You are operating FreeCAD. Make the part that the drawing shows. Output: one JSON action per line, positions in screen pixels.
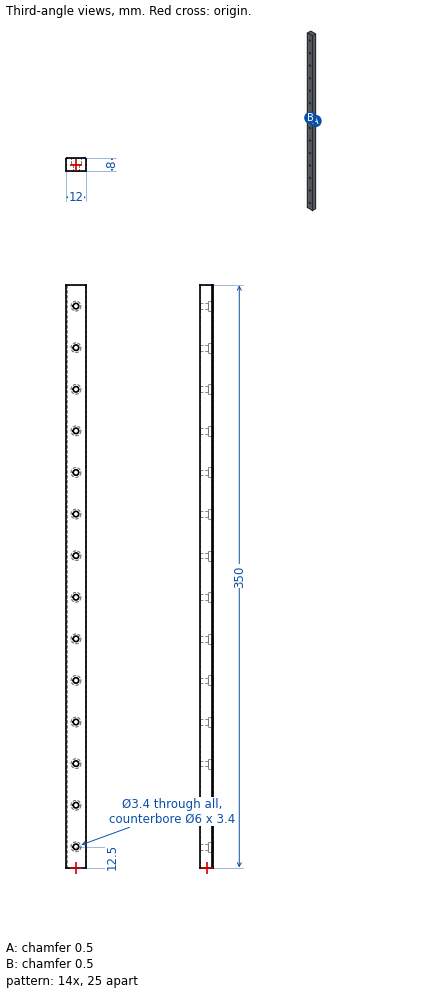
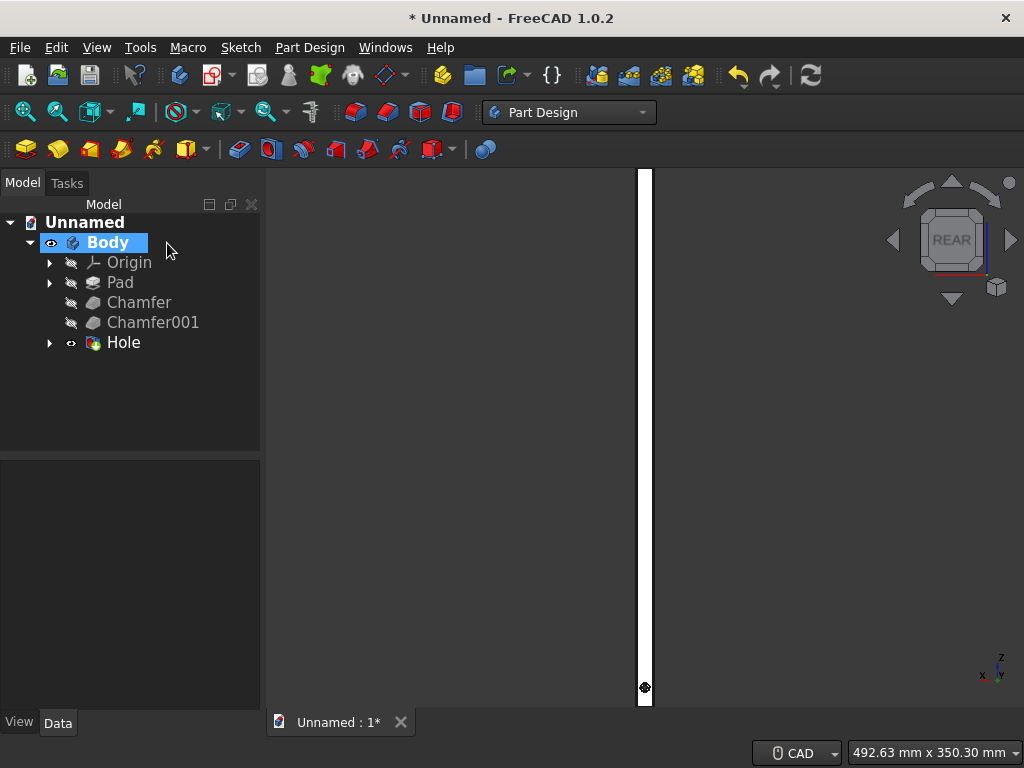
{"action": "left_click", "coordinate": [26, 112]}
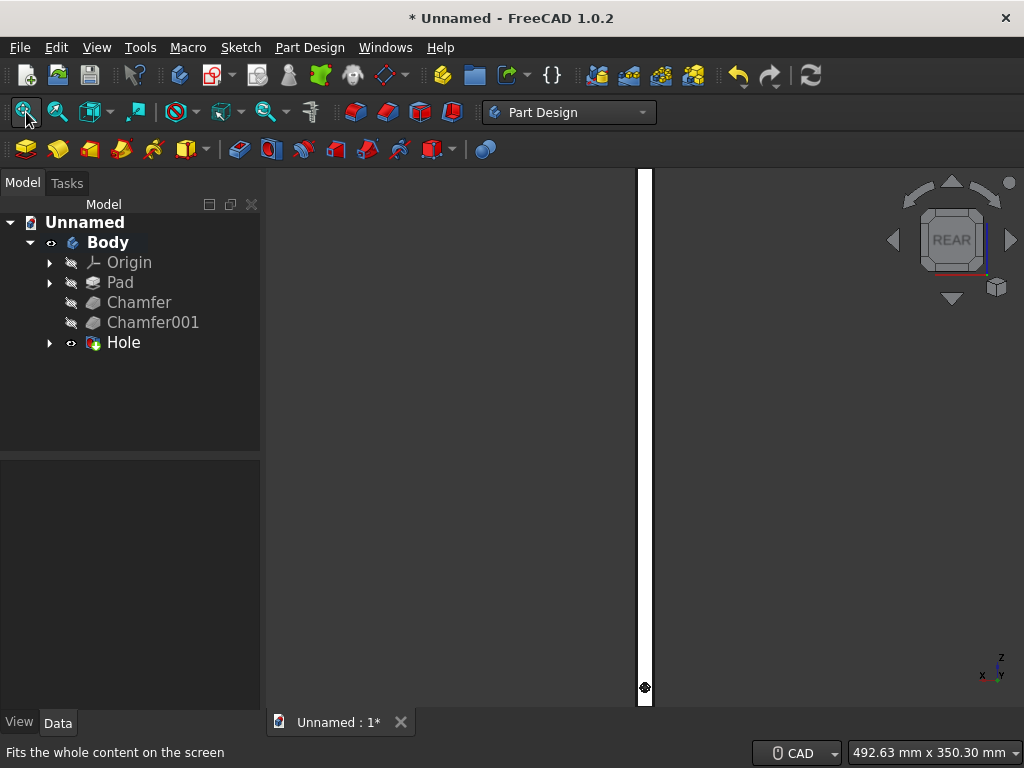
{"action": "left_click", "coordinate": [116, 343]}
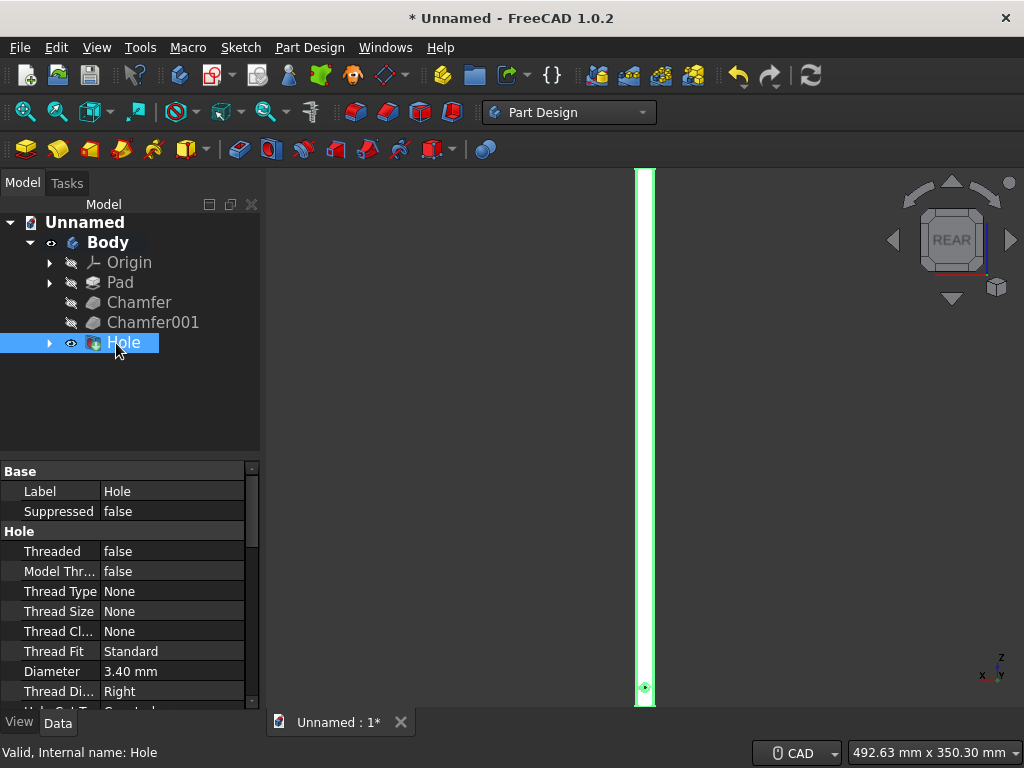
{"action": "left_click", "coordinate": [630, 76]}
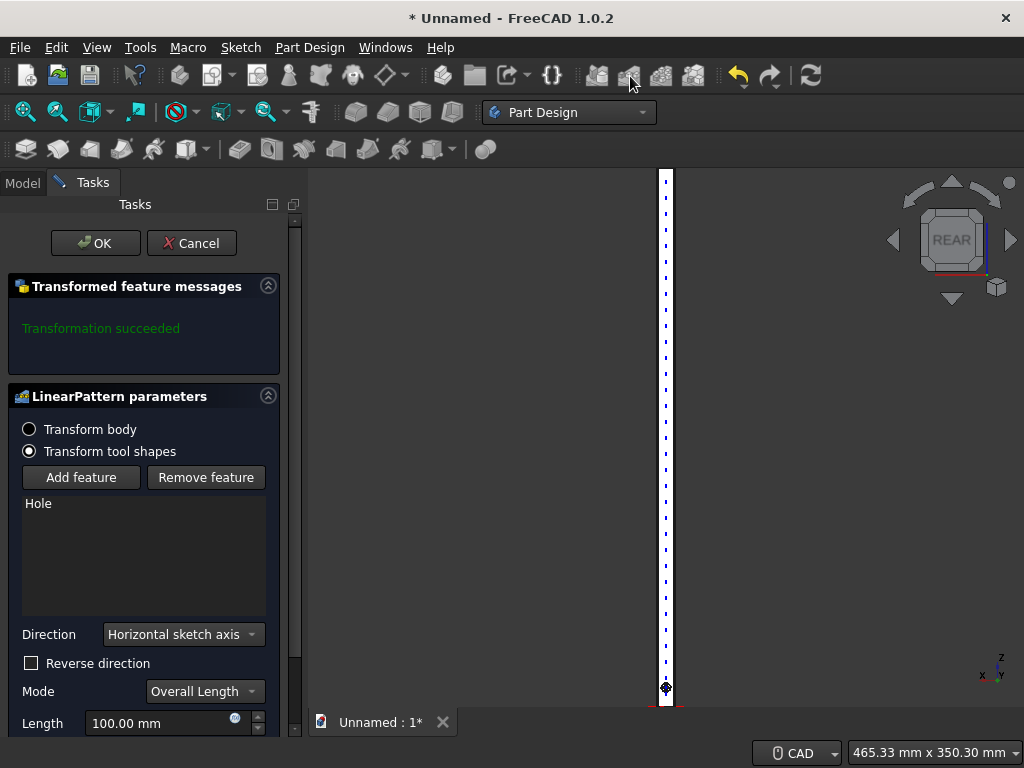
{"action": "left_click", "coordinate": [184, 634]}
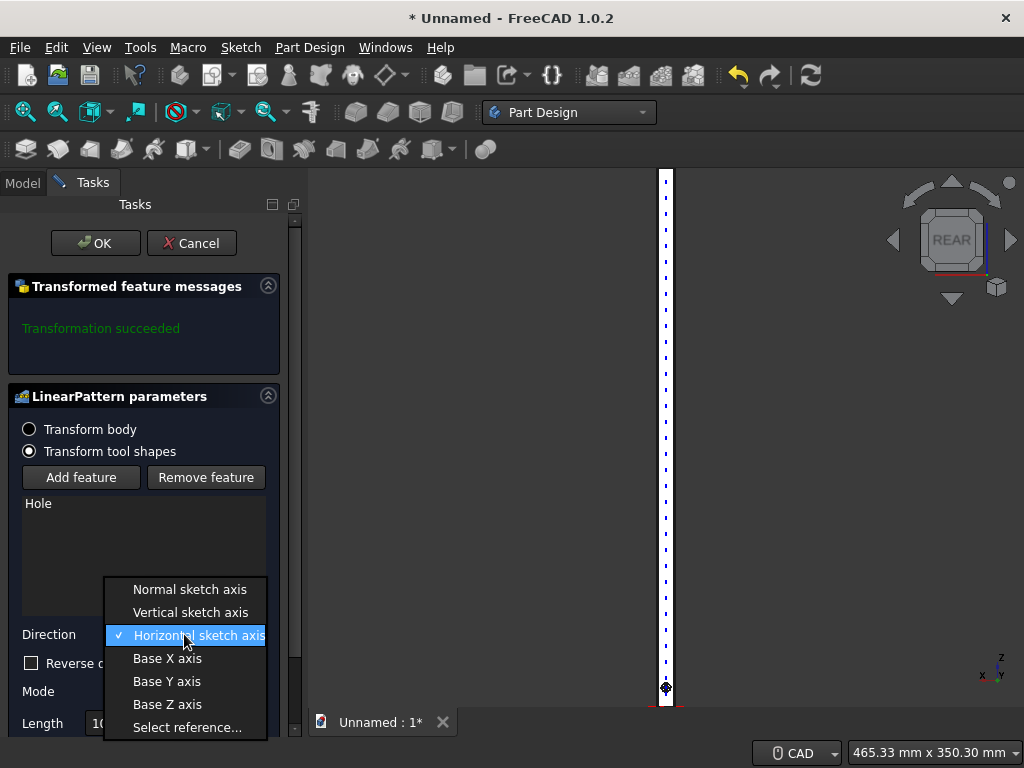
{"action": "left_click", "coordinate": [184, 704]}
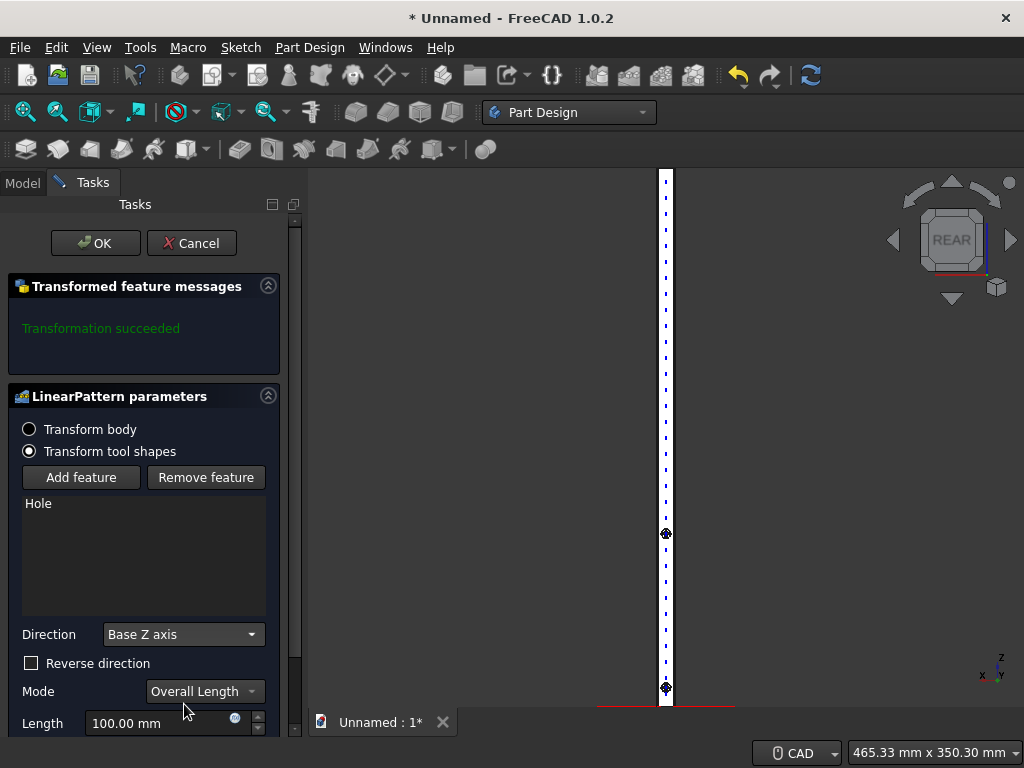
{"action": "left_click", "coordinate": [206, 692]}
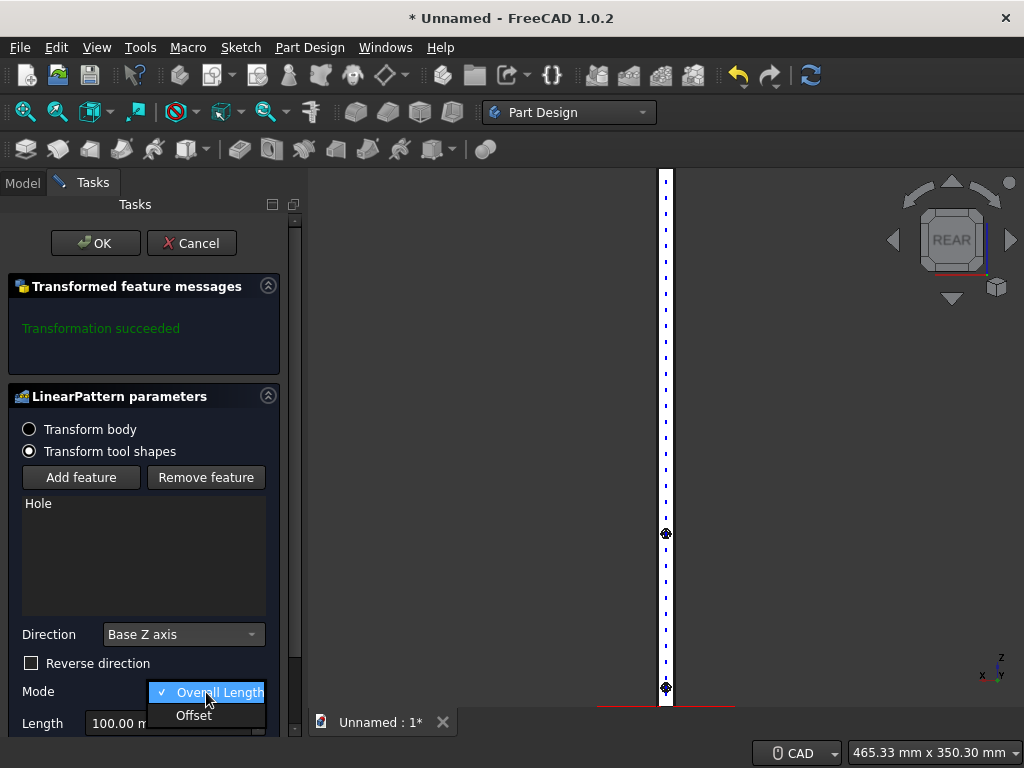
{"action": "left_click", "coordinate": [206, 716]}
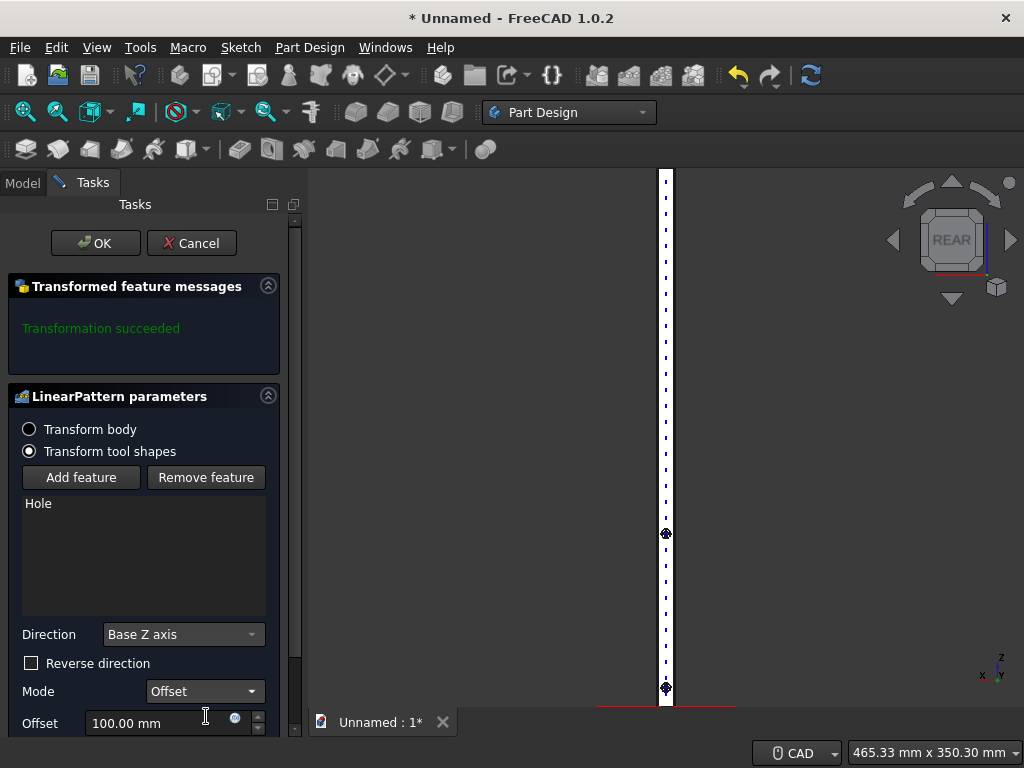
{"action": "triple_click", "coordinate": [168, 723]}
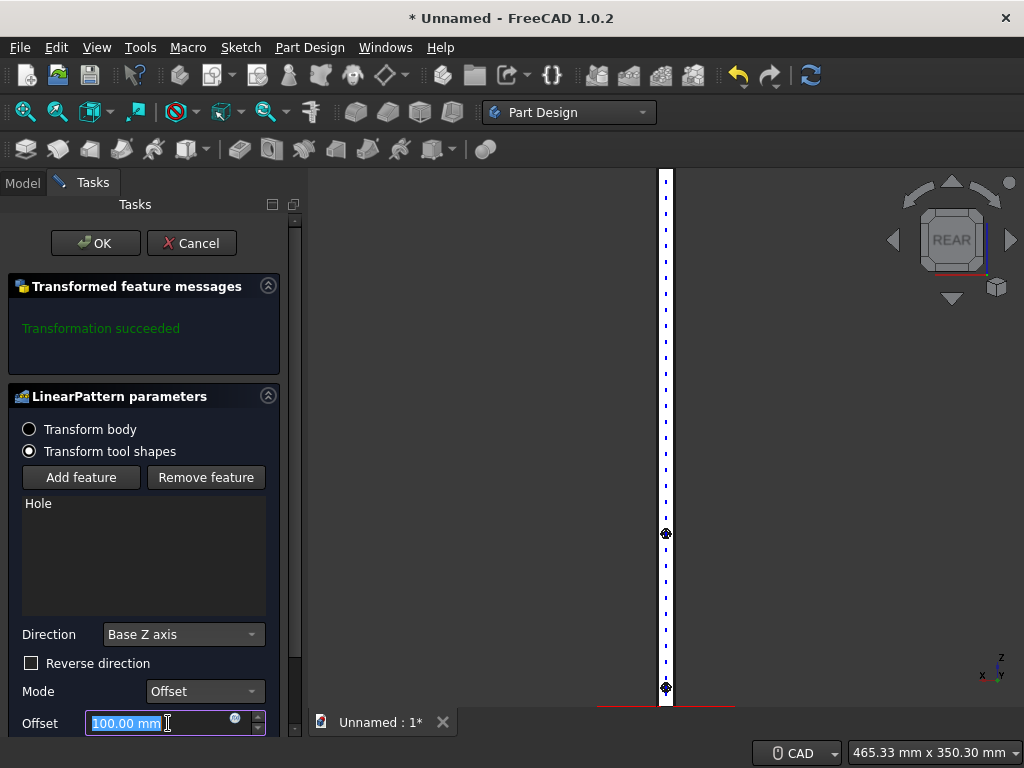
{"action": "type", "text": "25"}
{"action": "key", "text": "Tab"}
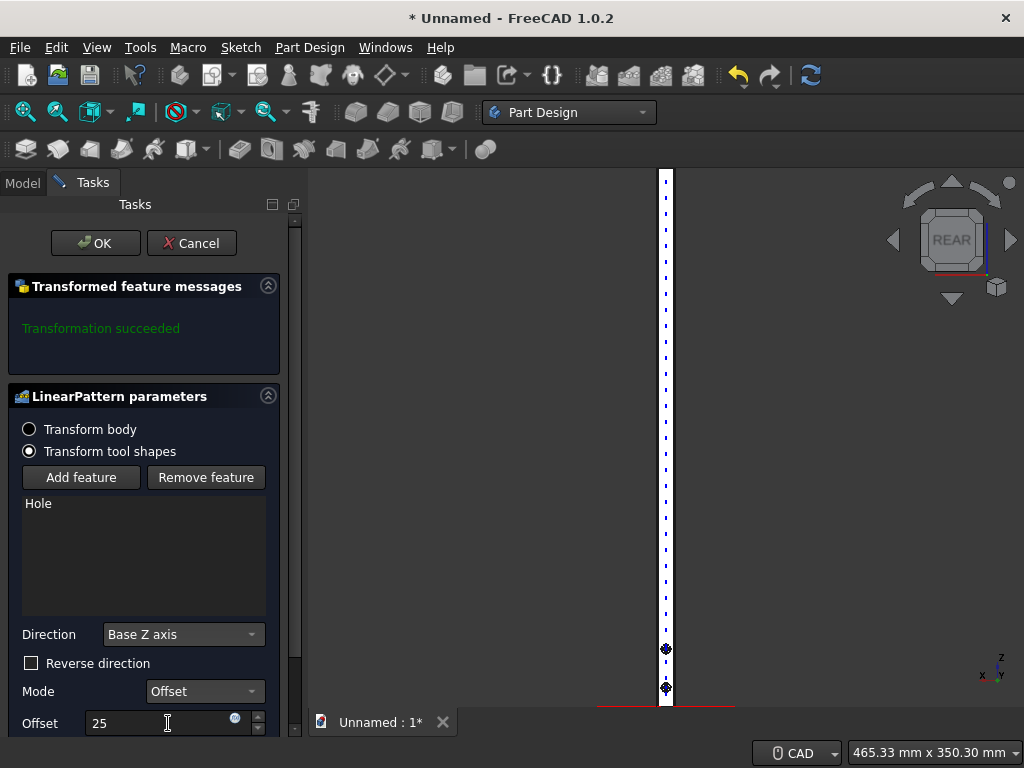
{"action": "scroll", "coordinate": [295, 475], "scroll_direction": "down", "scroll_amount": 2}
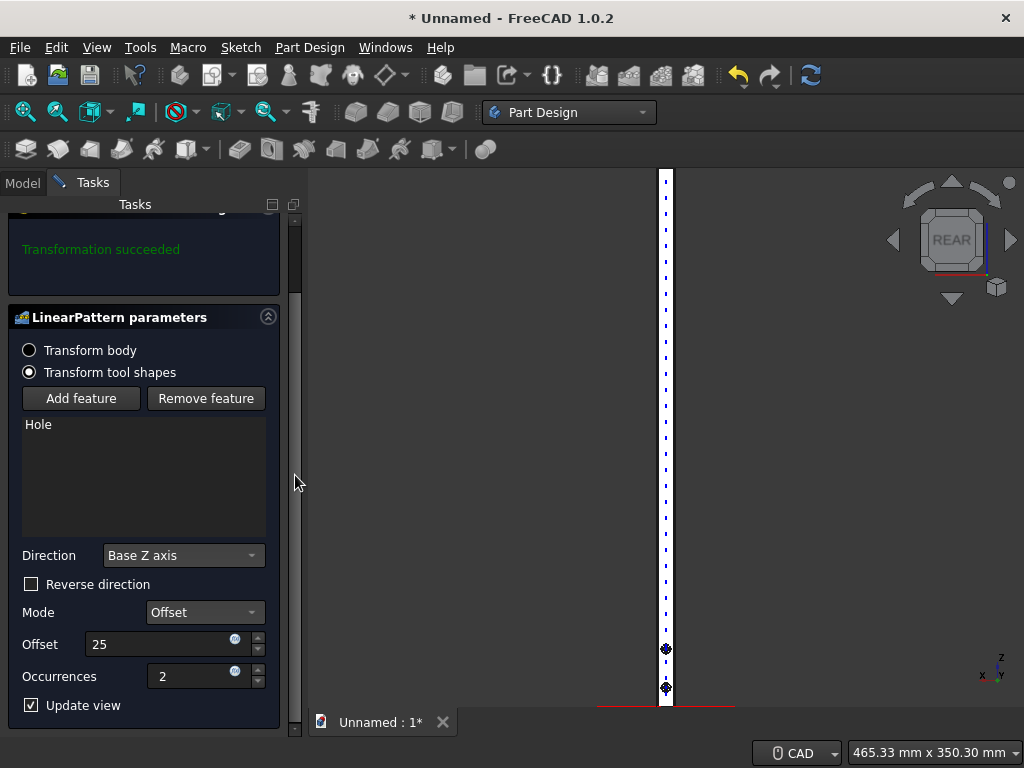
{"action": "triple_click", "coordinate": [198, 676]}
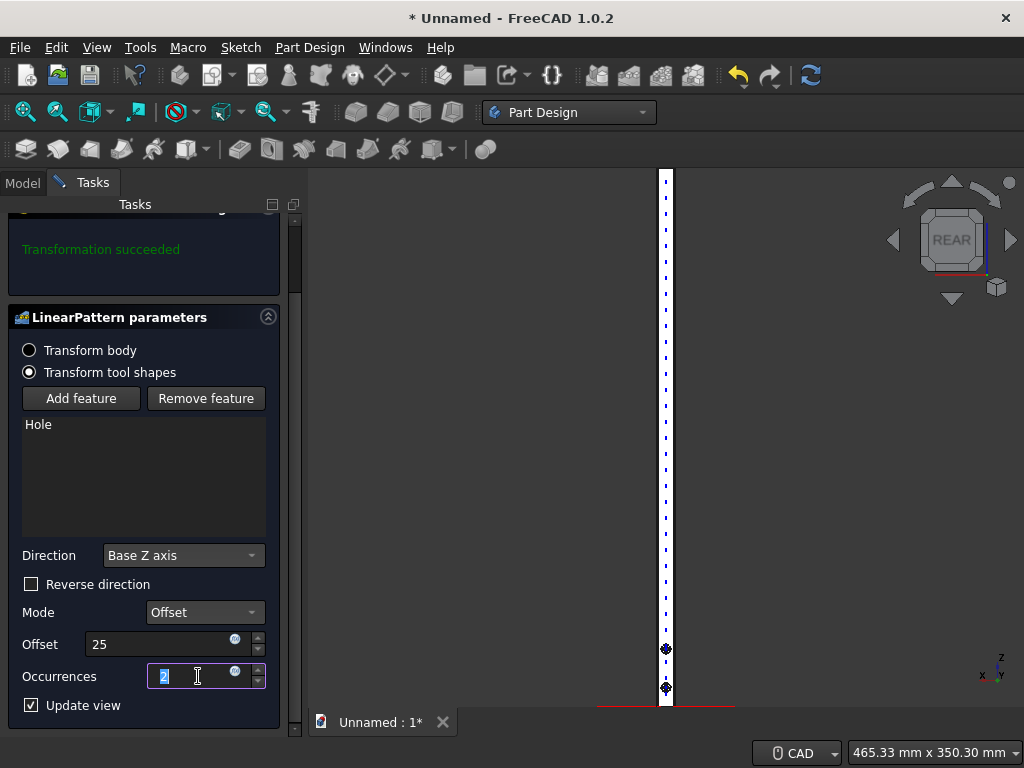
{"action": "type", "text": "14"}
{"action": "key", "text": "Tab"}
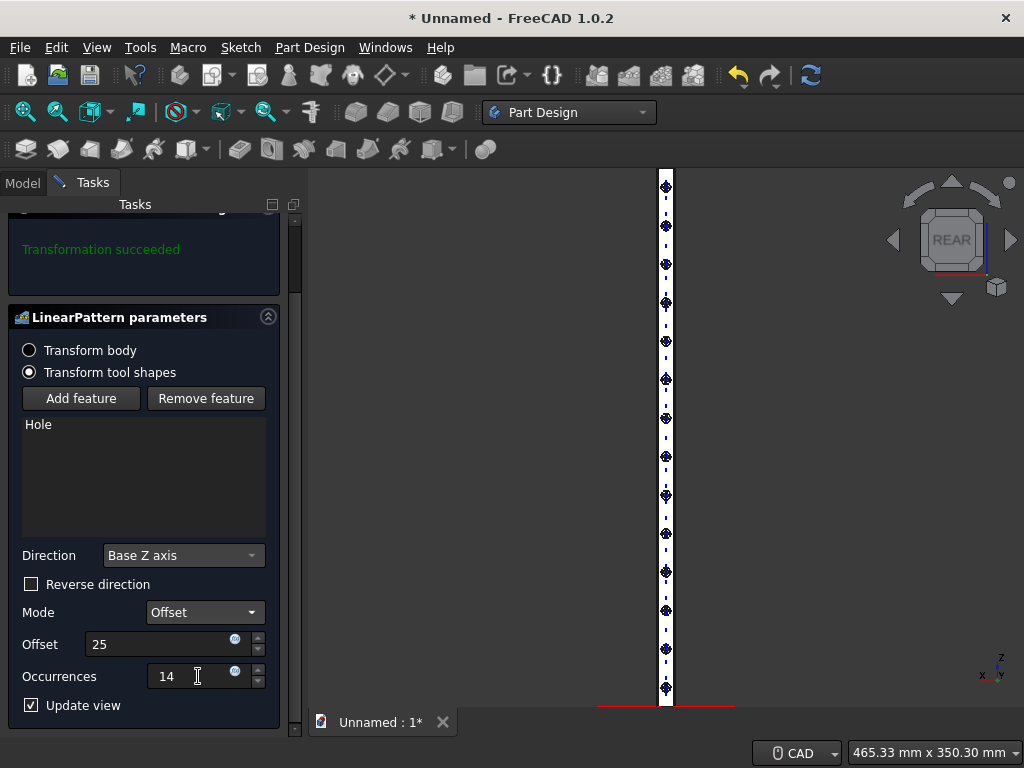
{"action": "scroll", "coordinate": [295, 475], "scroll_direction": "up", "scroll_amount": 3}